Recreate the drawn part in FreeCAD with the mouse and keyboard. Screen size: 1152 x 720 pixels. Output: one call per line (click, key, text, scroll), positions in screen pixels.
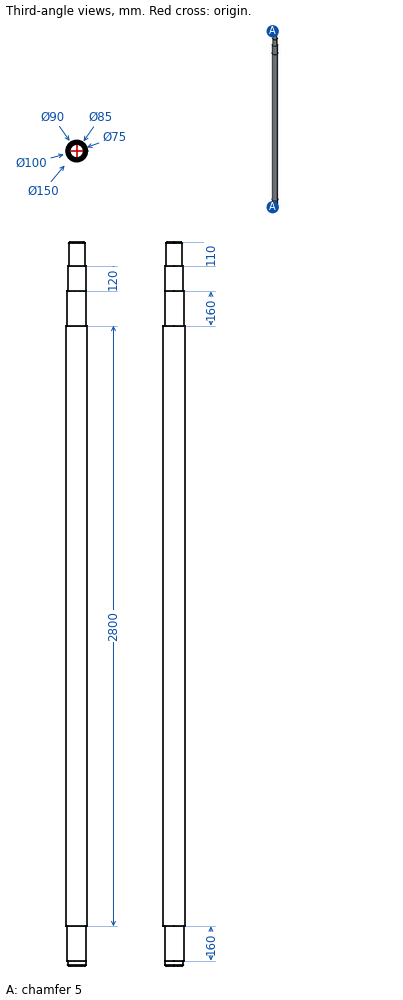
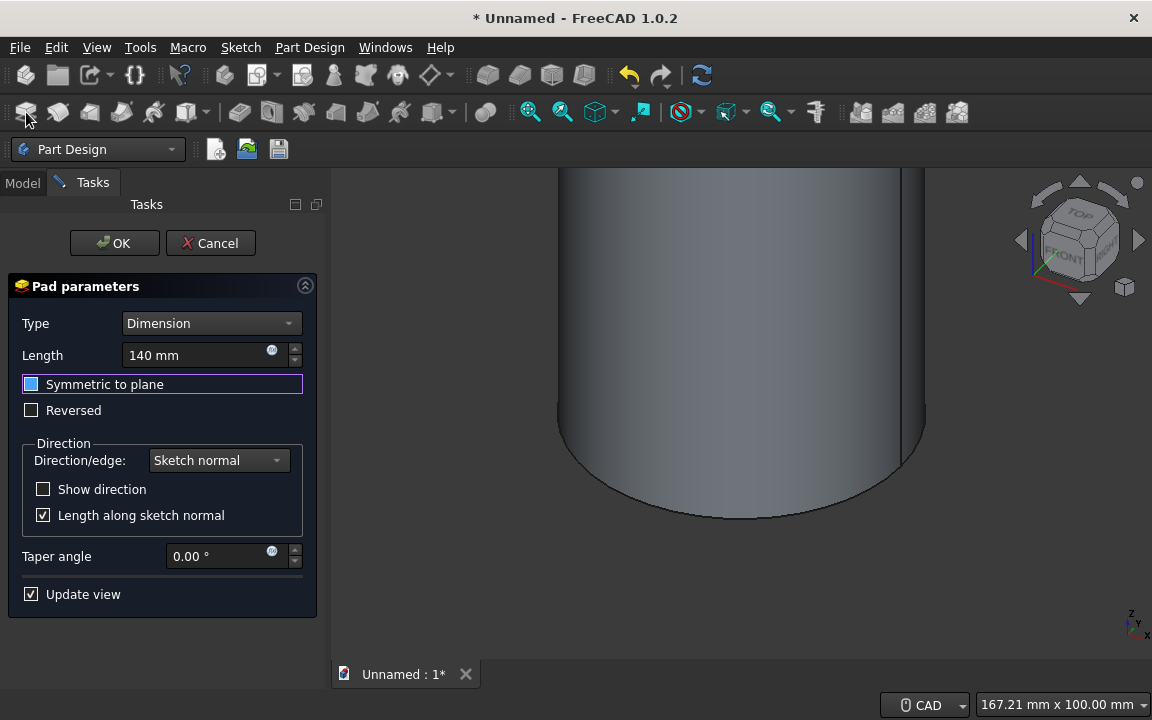
click(115, 243)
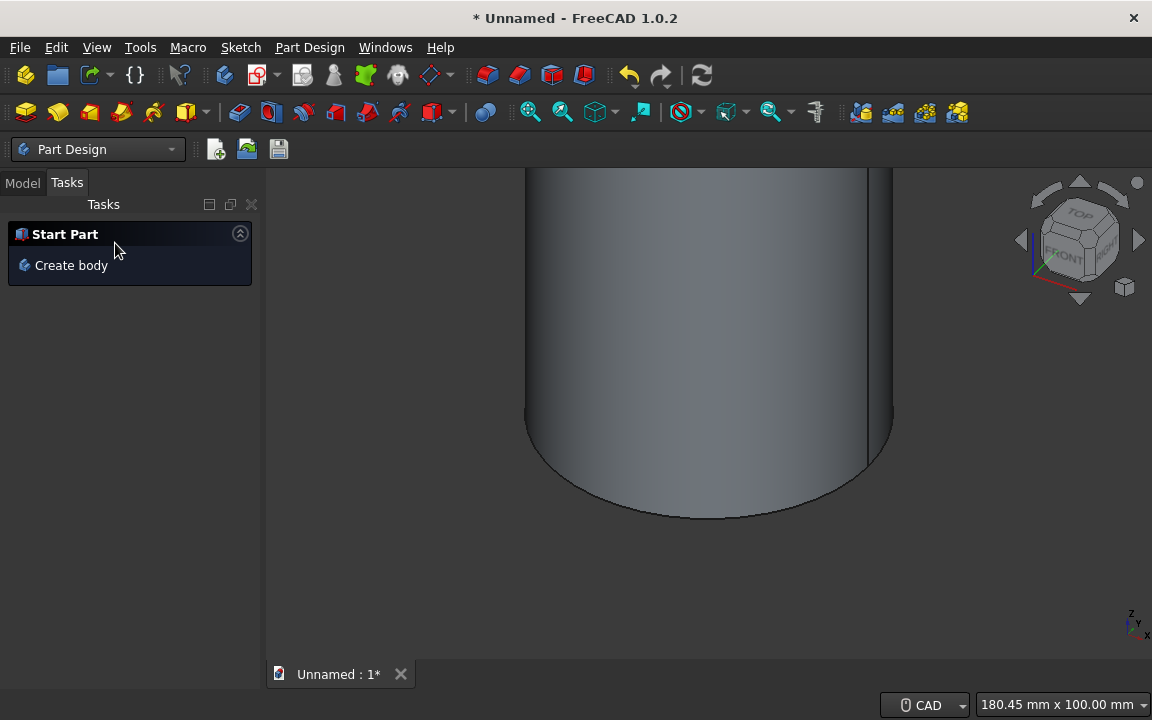
click(532, 112)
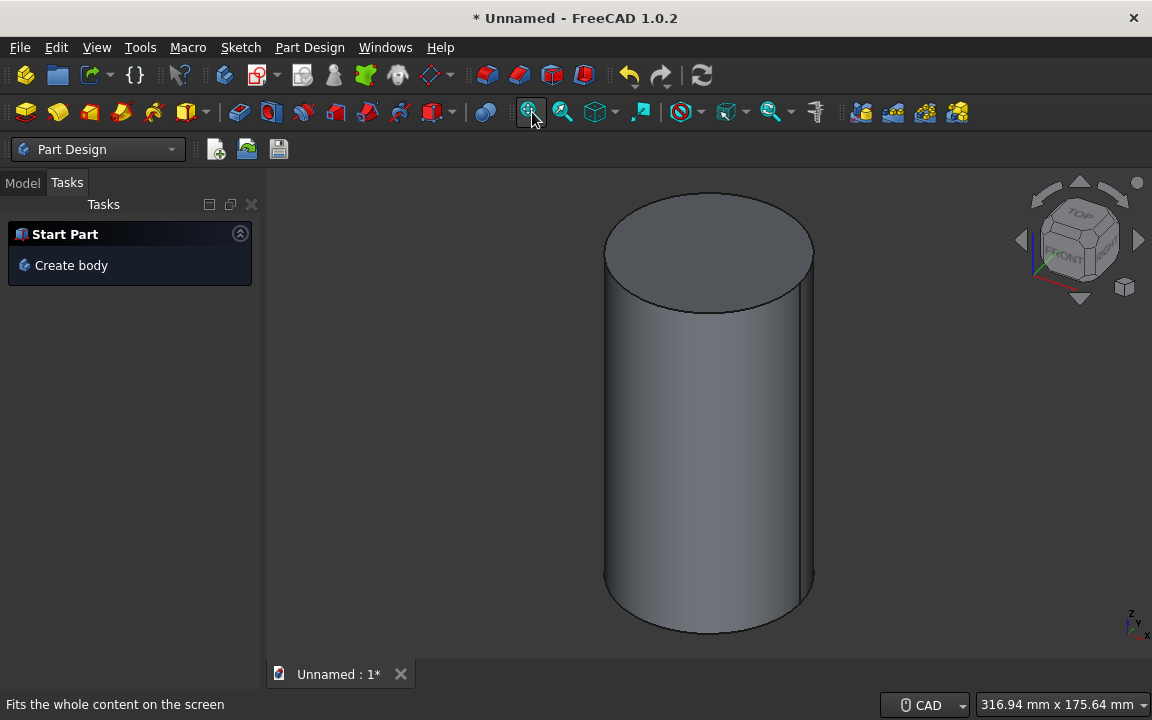
click(709, 252)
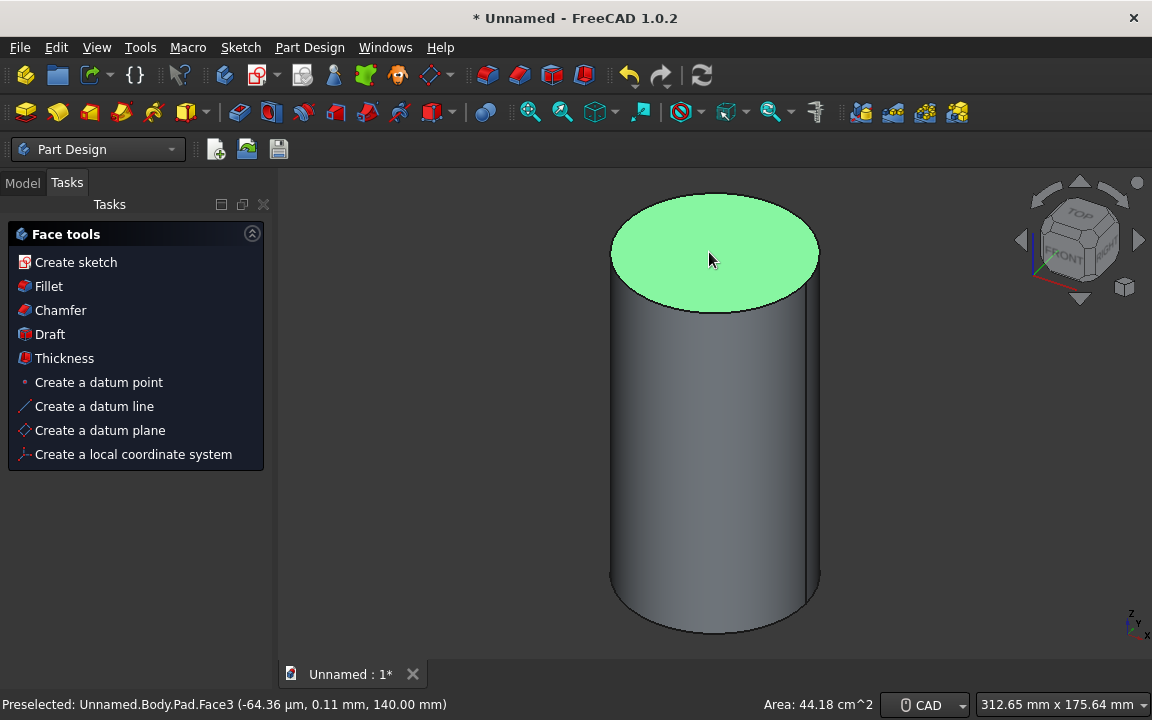
click(258, 76)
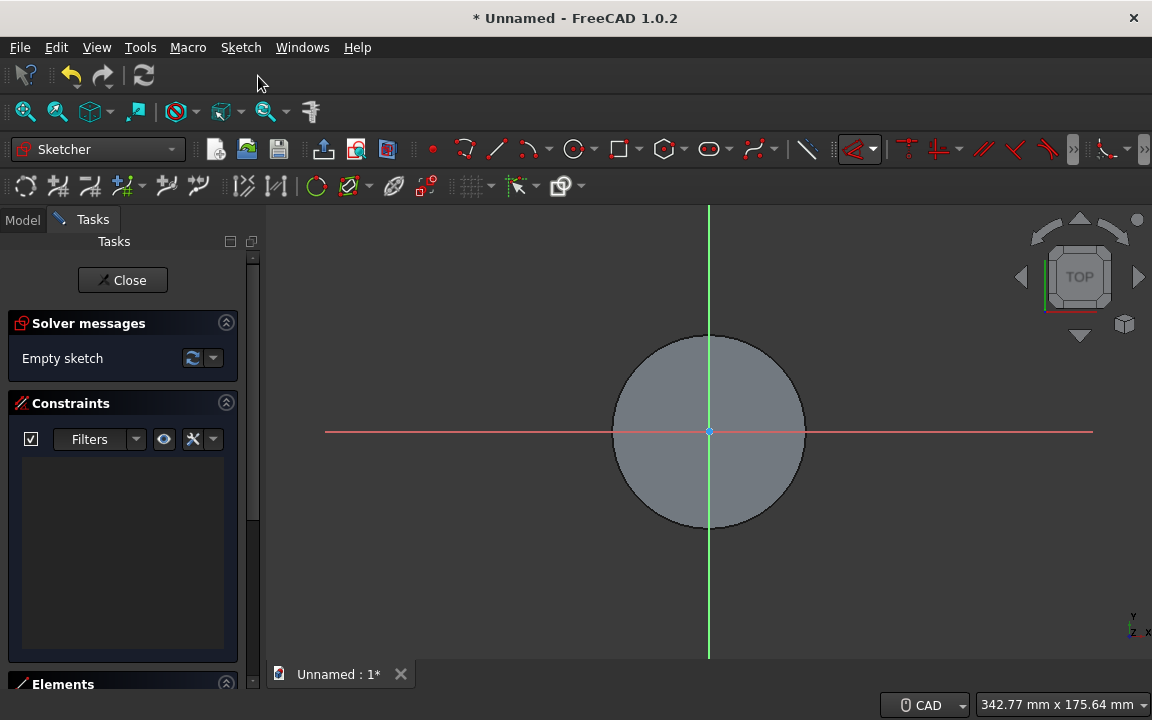
click(574, 150)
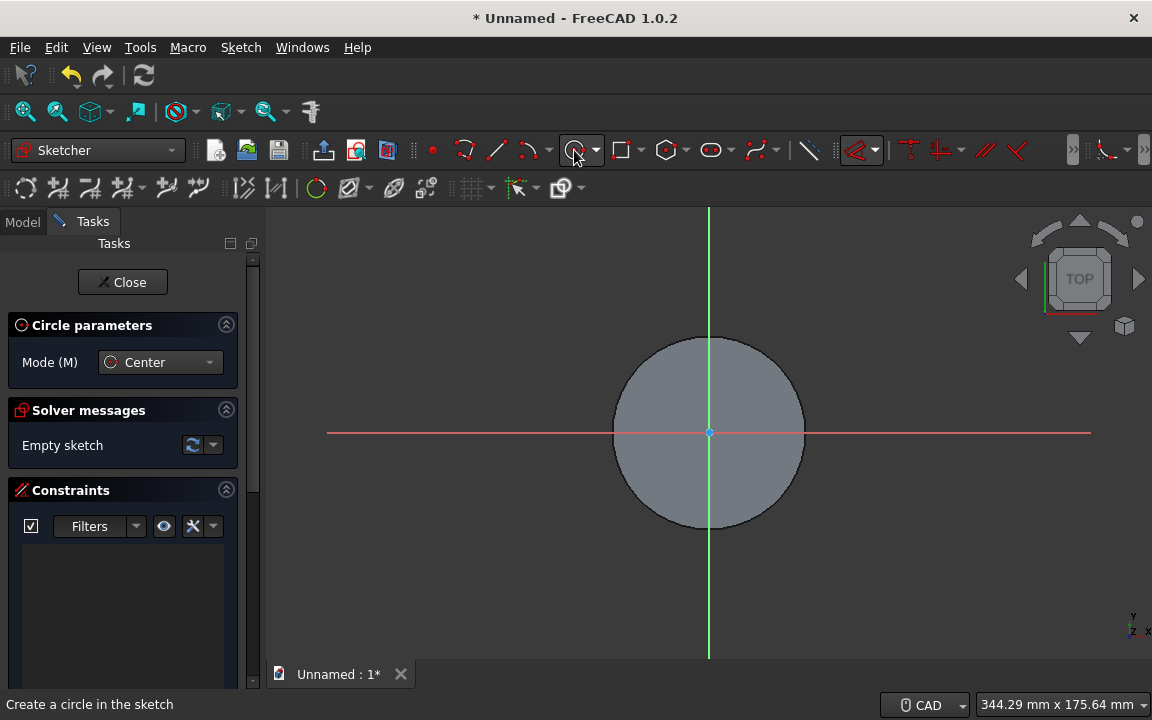
click(709, 433)
click(786, 356)
key(Escape)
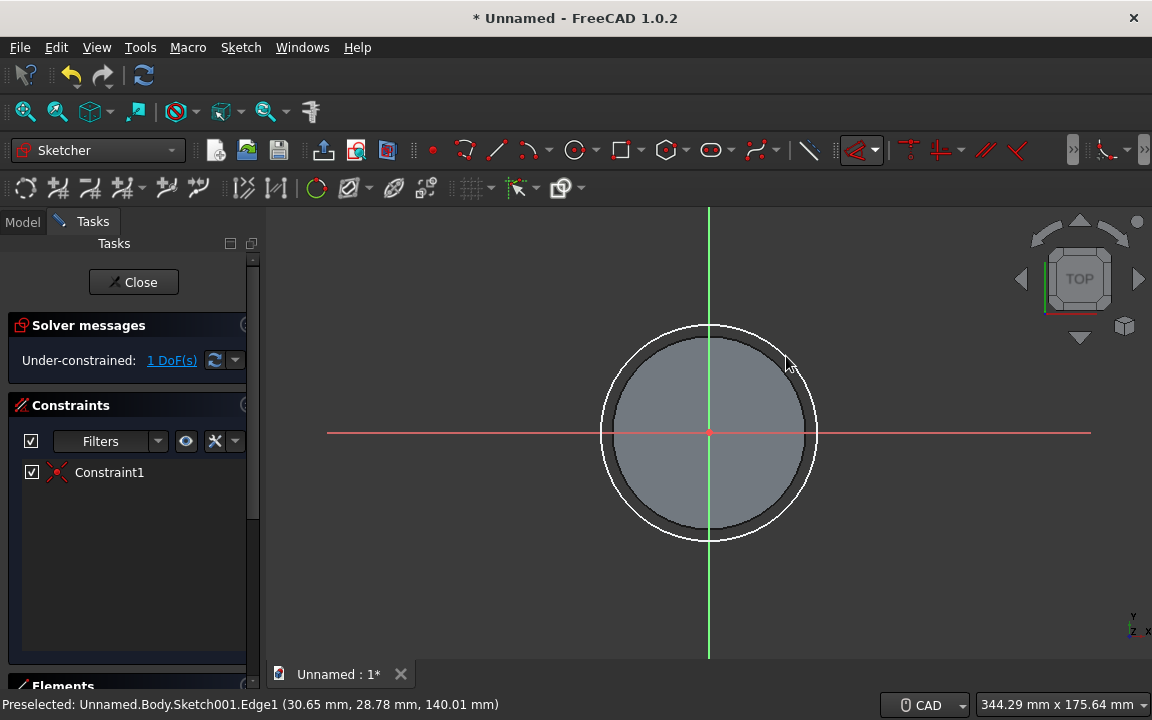
click(785, 356)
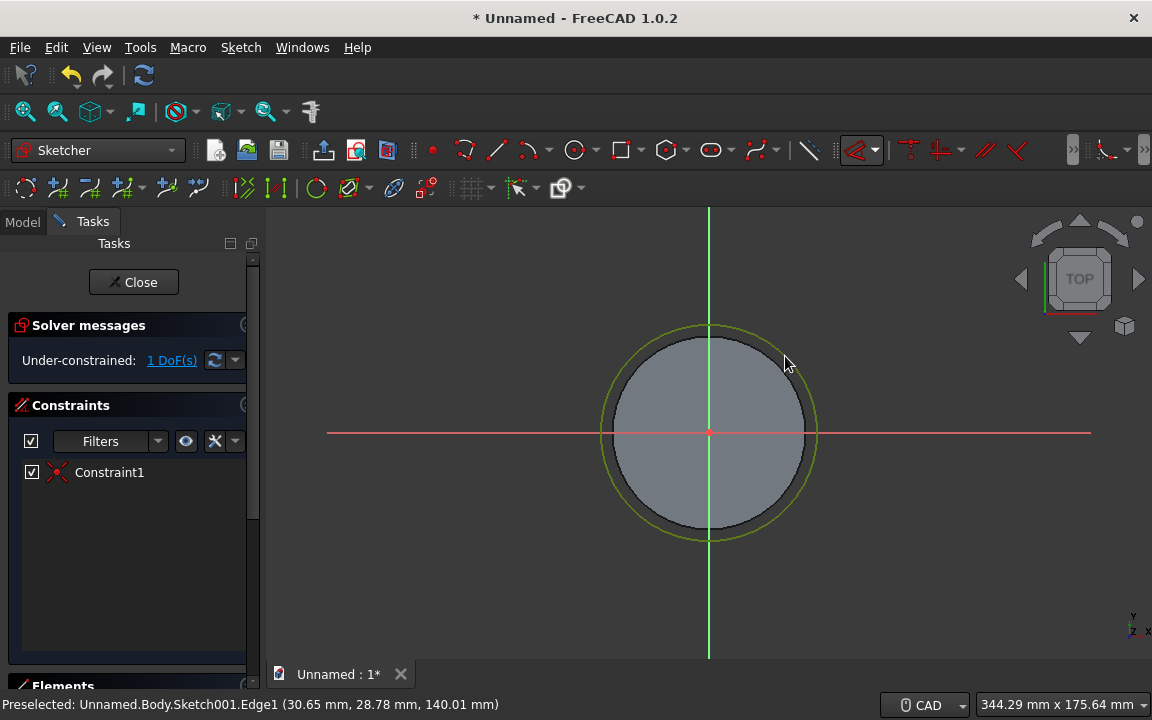
key(k)
key(o)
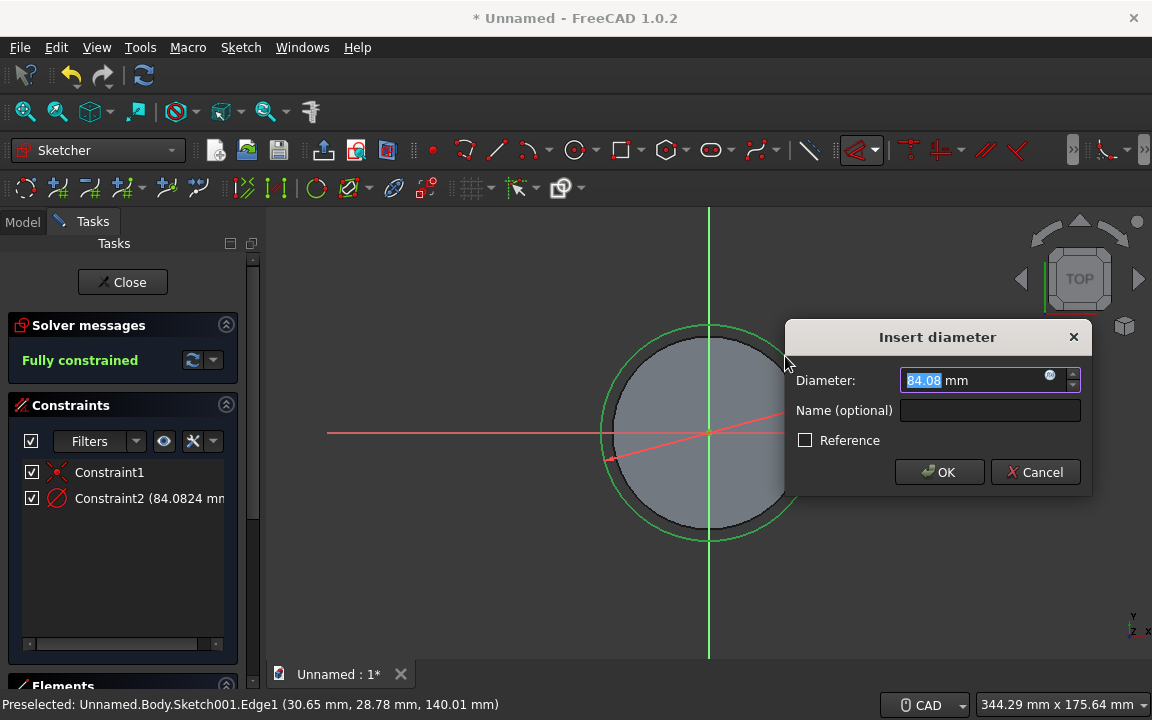
text(85)
key(Return)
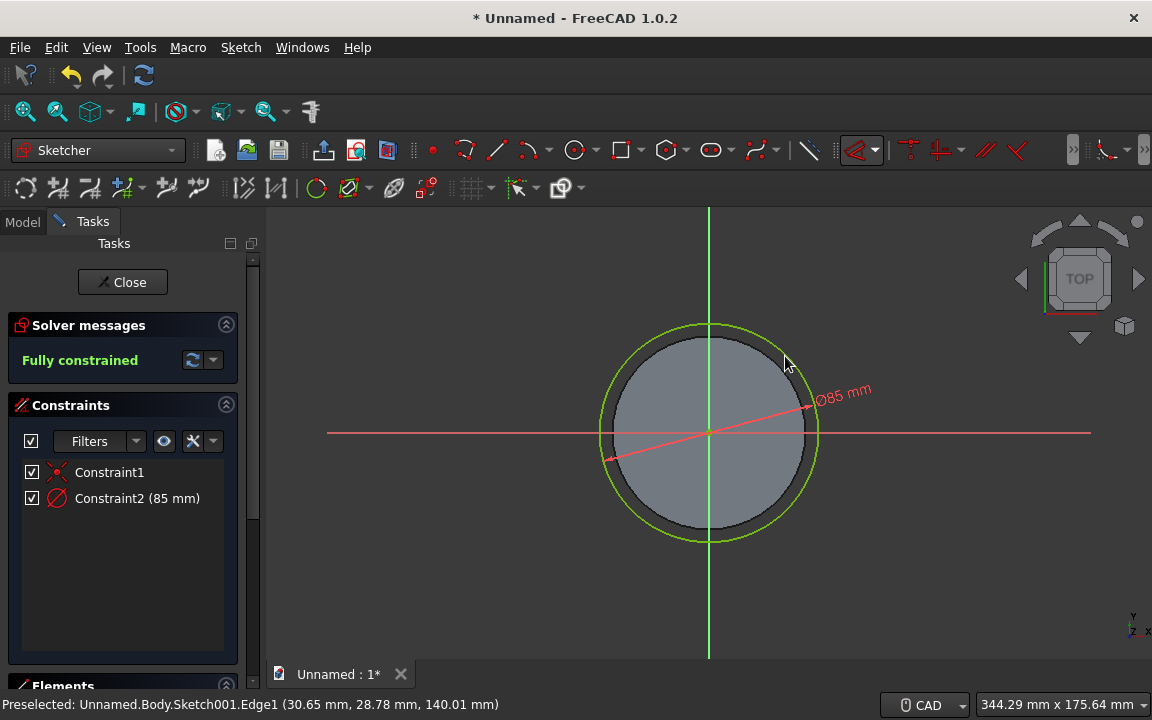
click(123, 282)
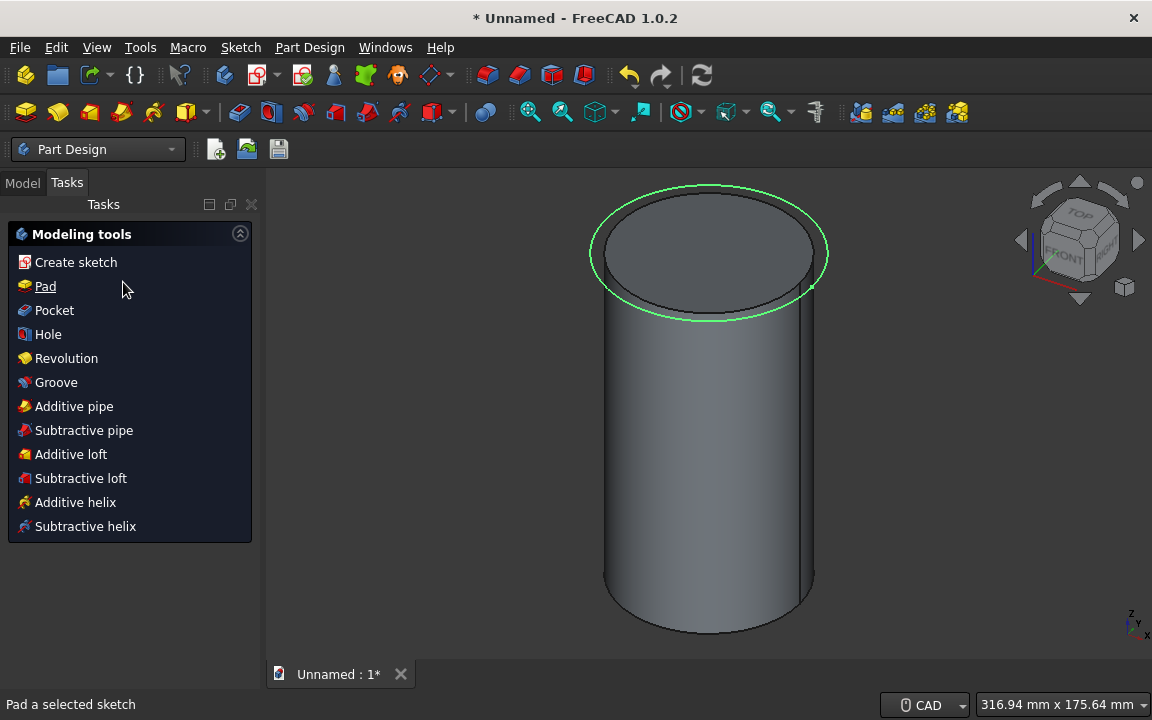
click(26, 112)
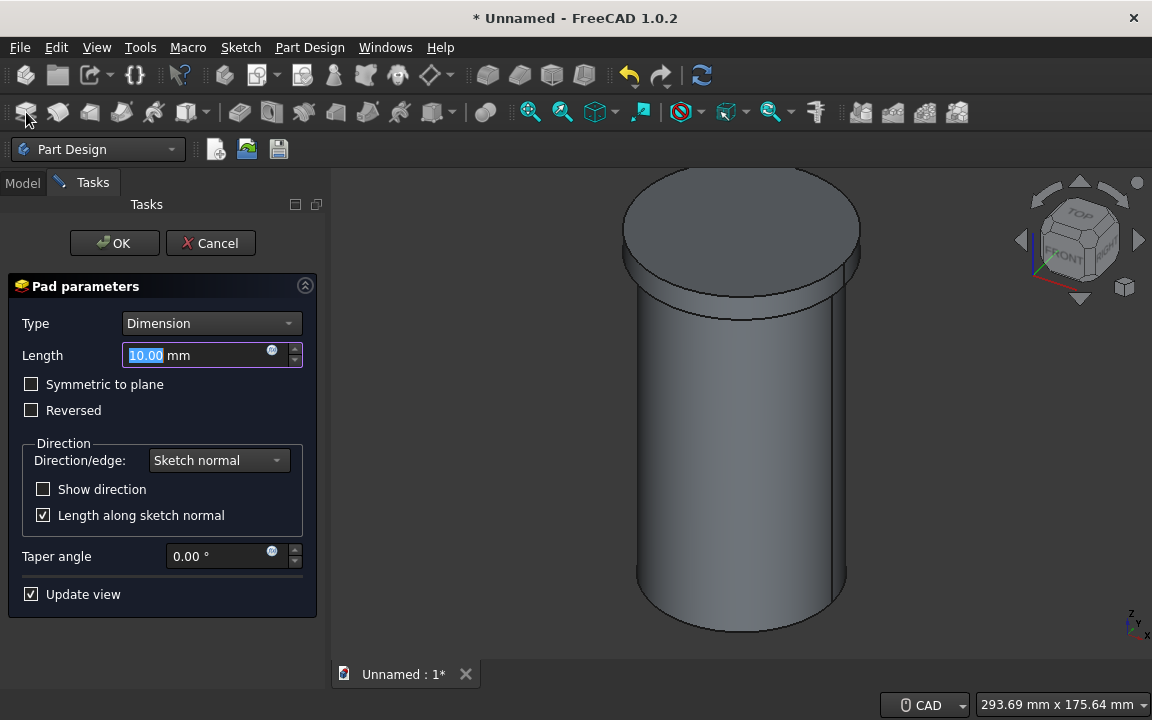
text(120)
key(Tab)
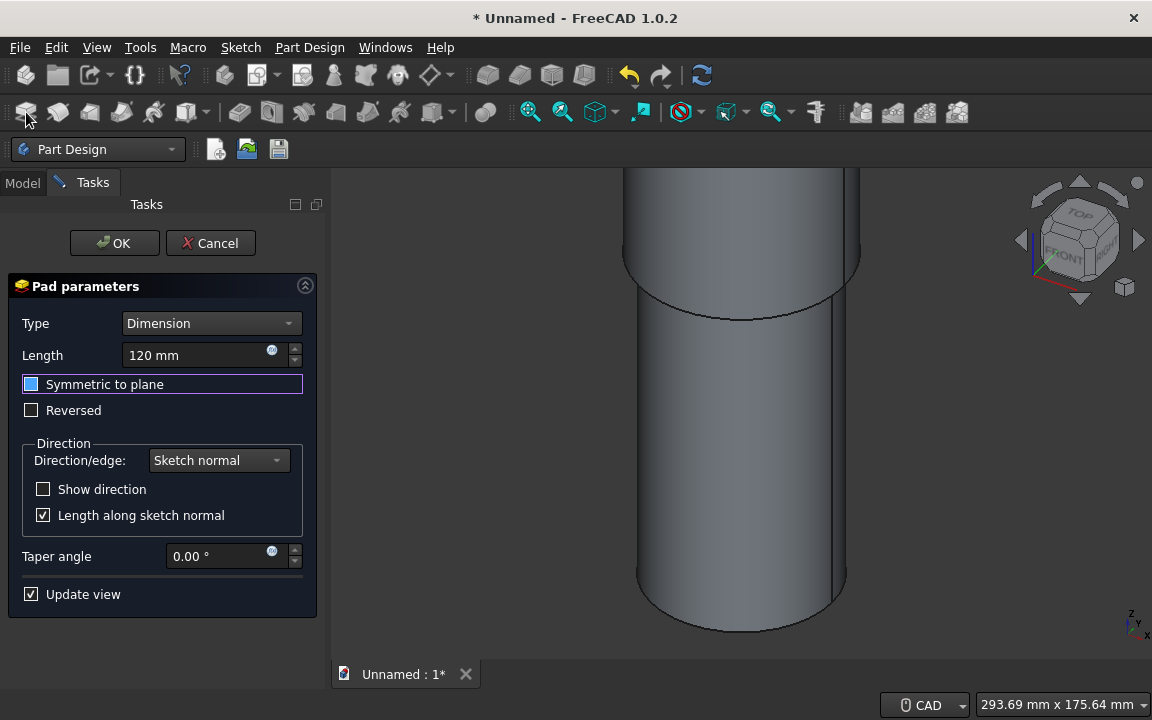
click(115, 243)